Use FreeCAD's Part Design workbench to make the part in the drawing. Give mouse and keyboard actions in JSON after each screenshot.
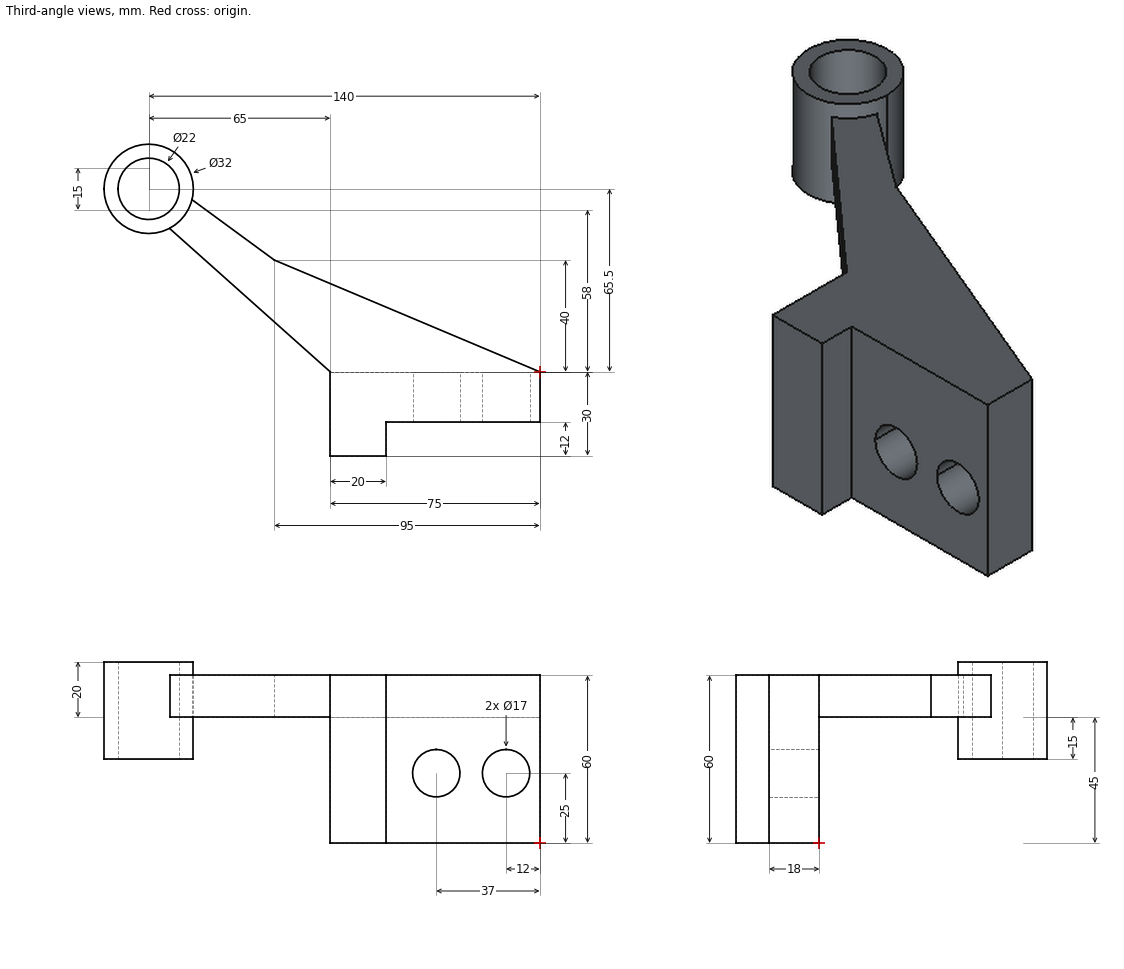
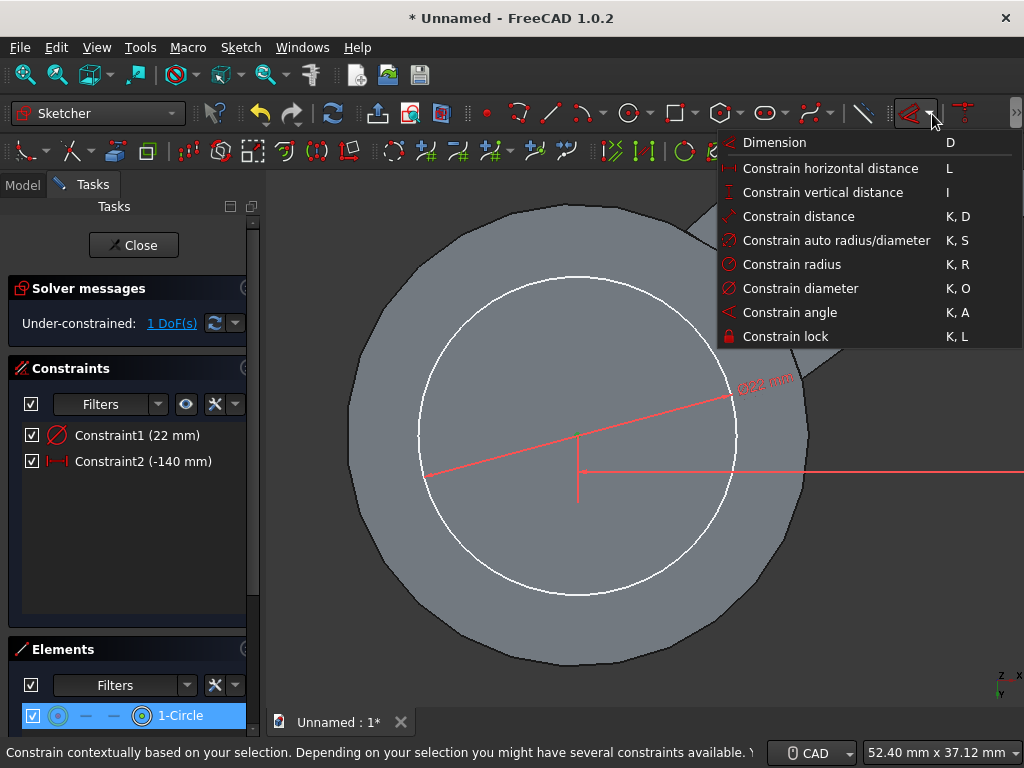
{"action": "left_click", "coordinate": [870, 192]}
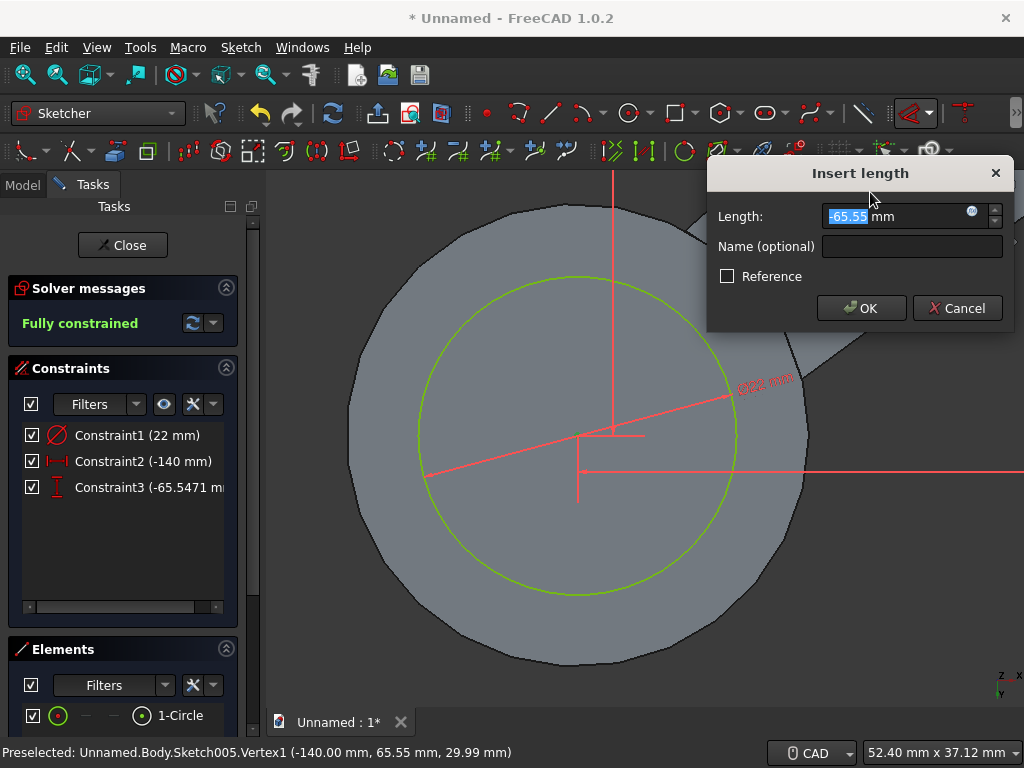
{"action": "type", "text": "-65.5"}
{"action": "key", "text": "Return"}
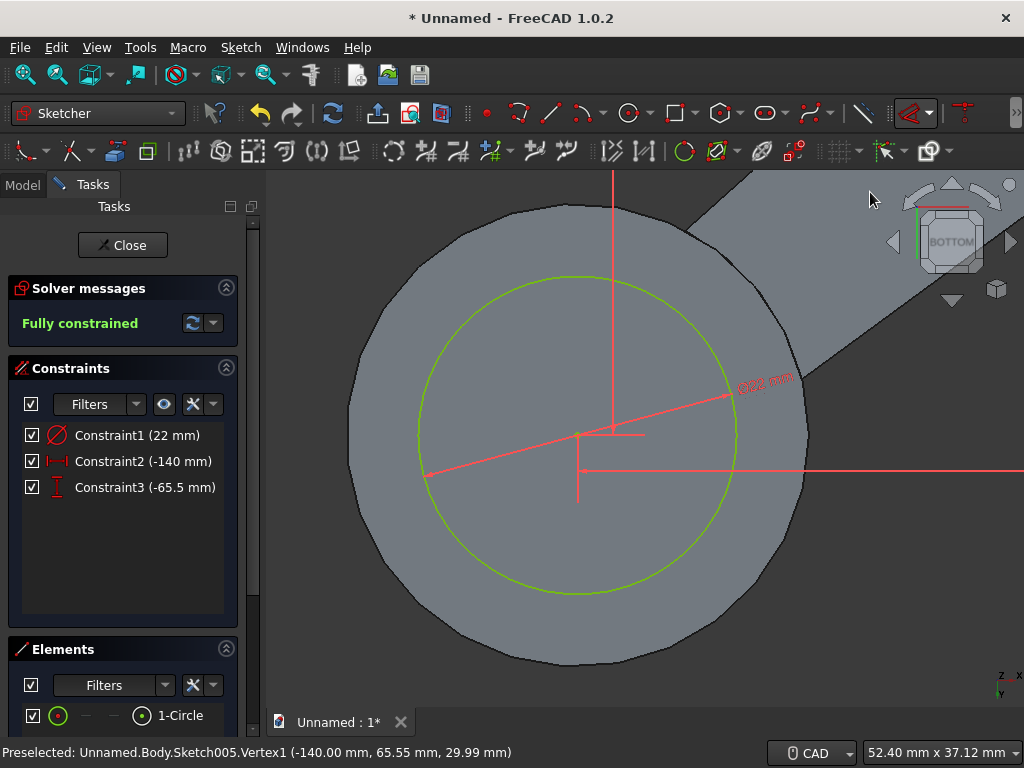
{"action": "left_click", "coordinate": [123, 245]}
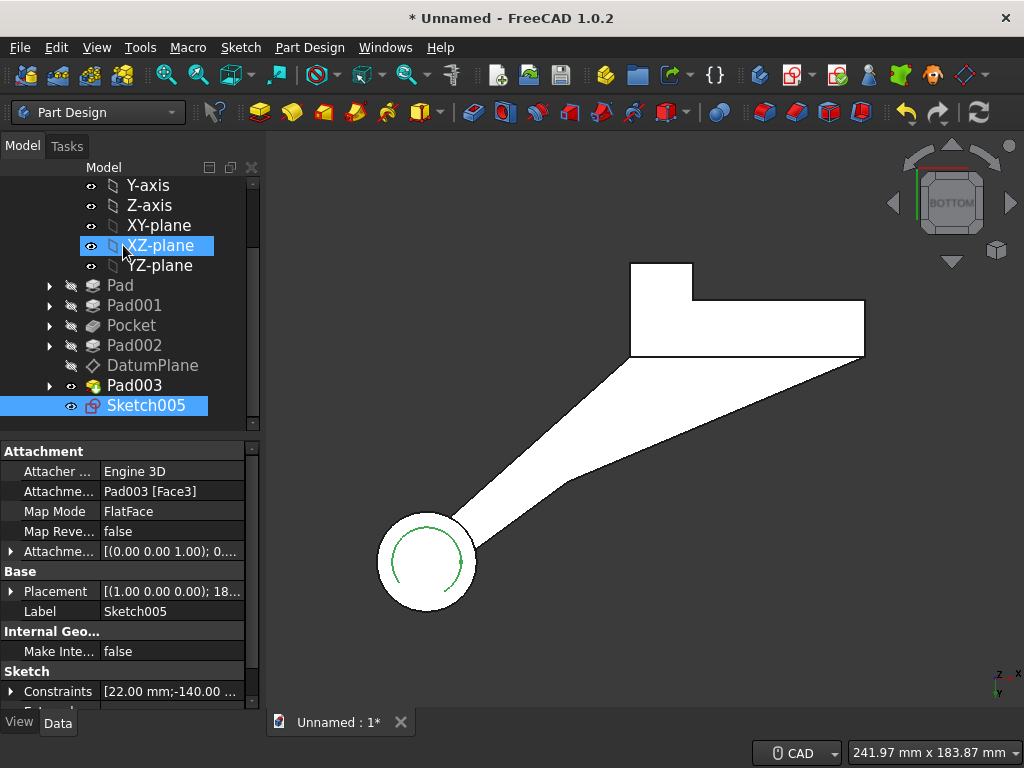
{"action": "left_click", "coordinate": [474, 112]}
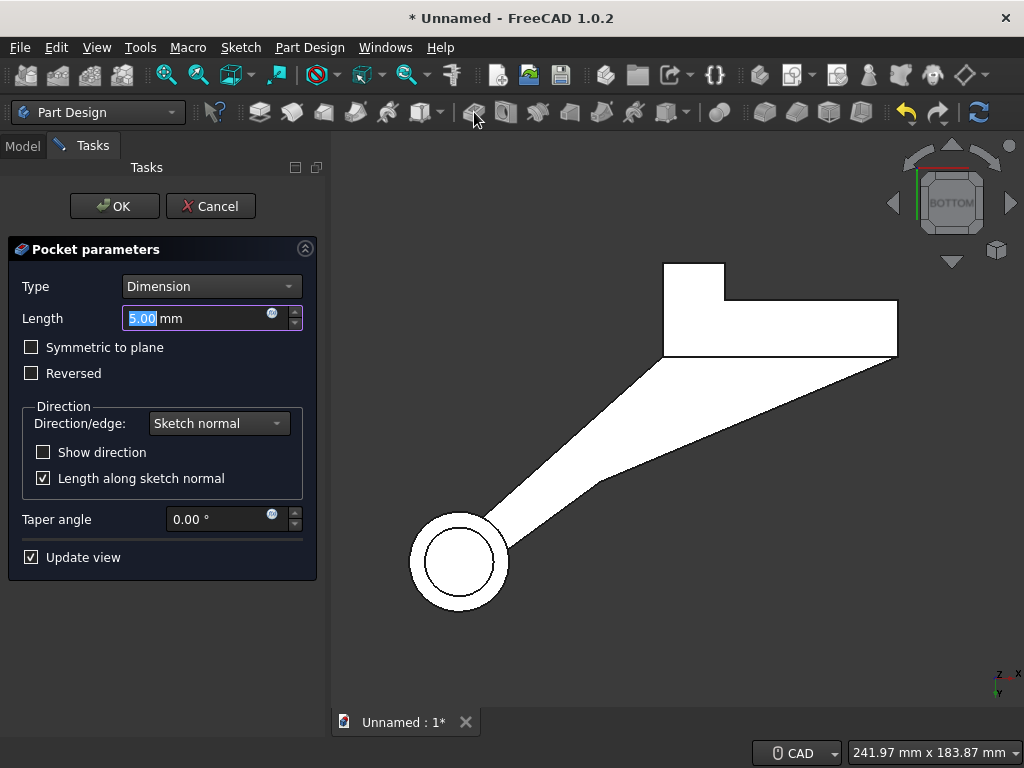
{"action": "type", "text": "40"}
{"action": "key", "text": "Tab"}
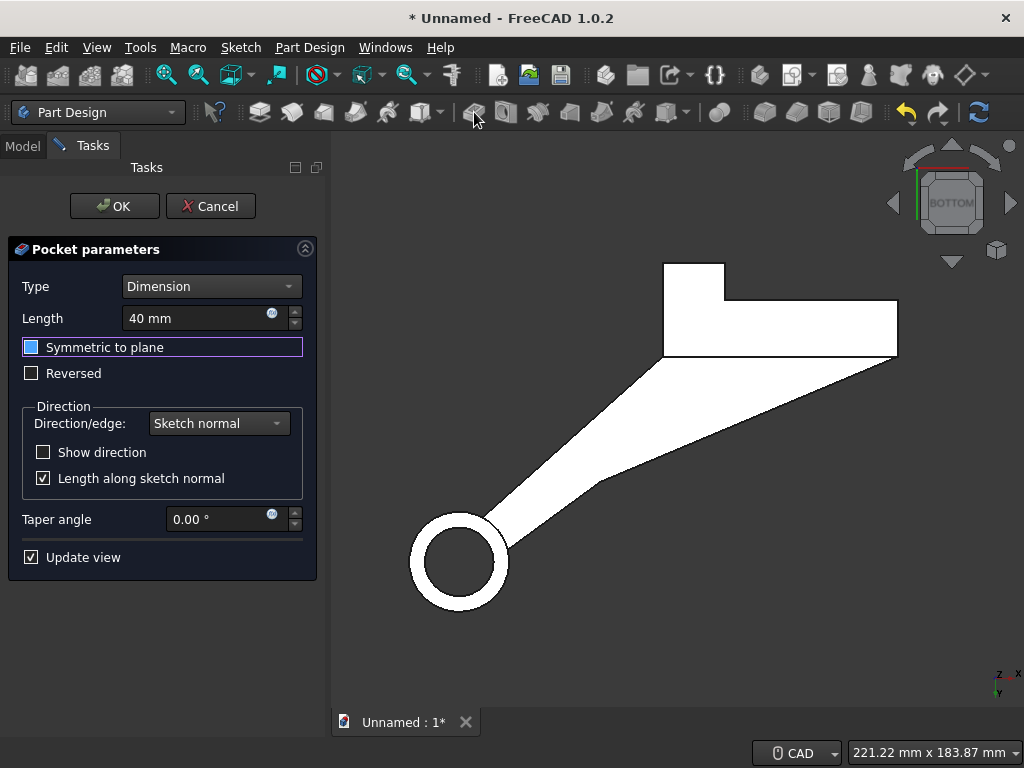
{"action": "left_click", "coordinate": [115, 206]}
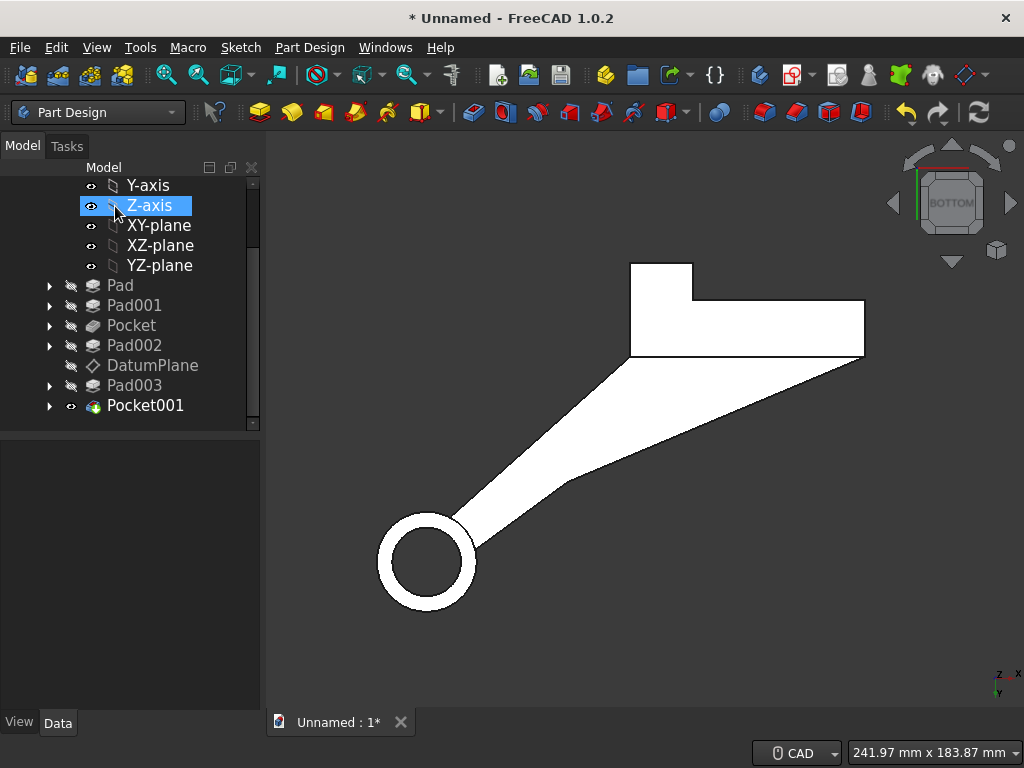
{"action": "key", "text": "4"}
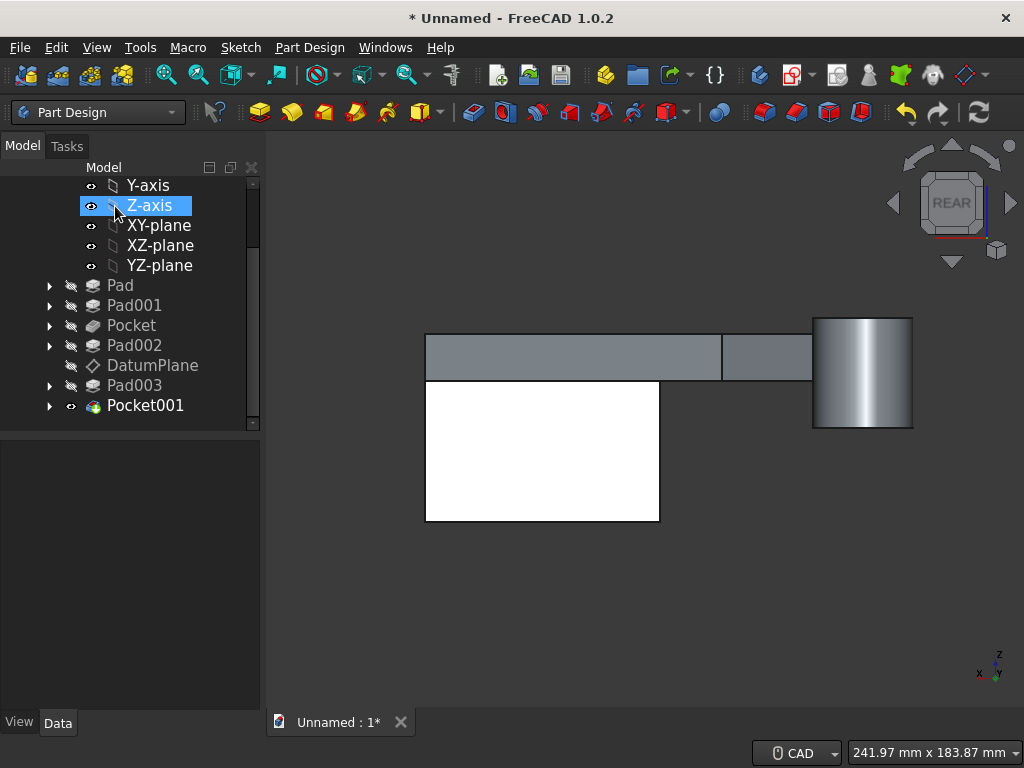
{"action": "left_click", "coordinate": [509, 450]}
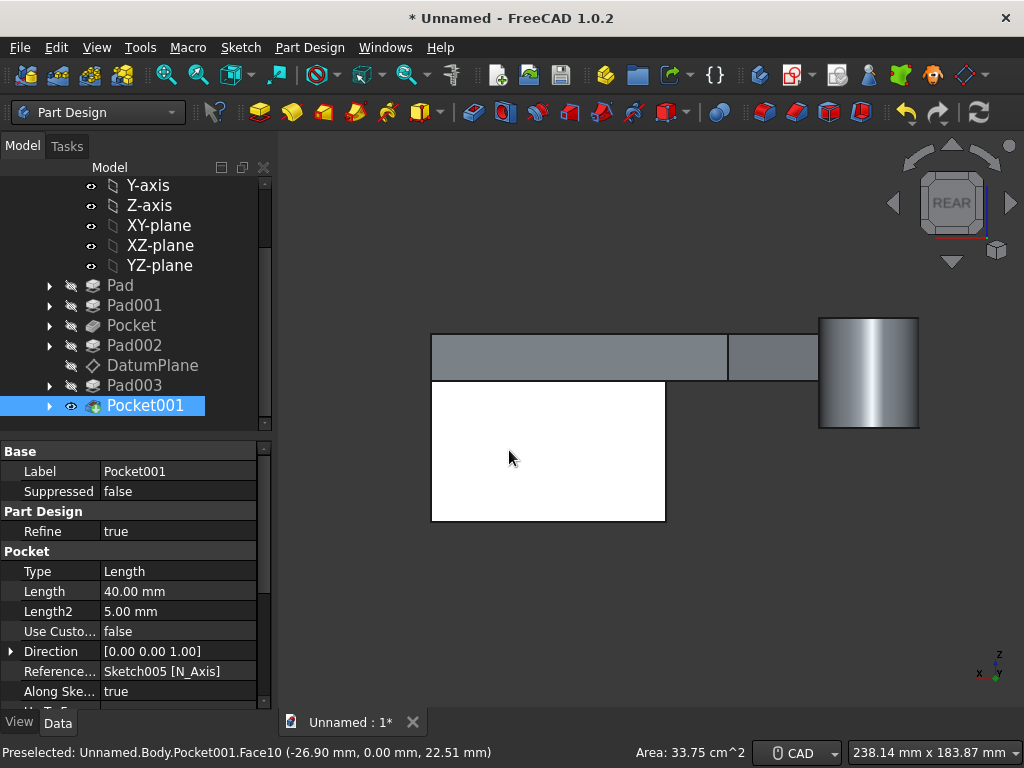
{"action": "left_click", "coordinate": [792, 76]}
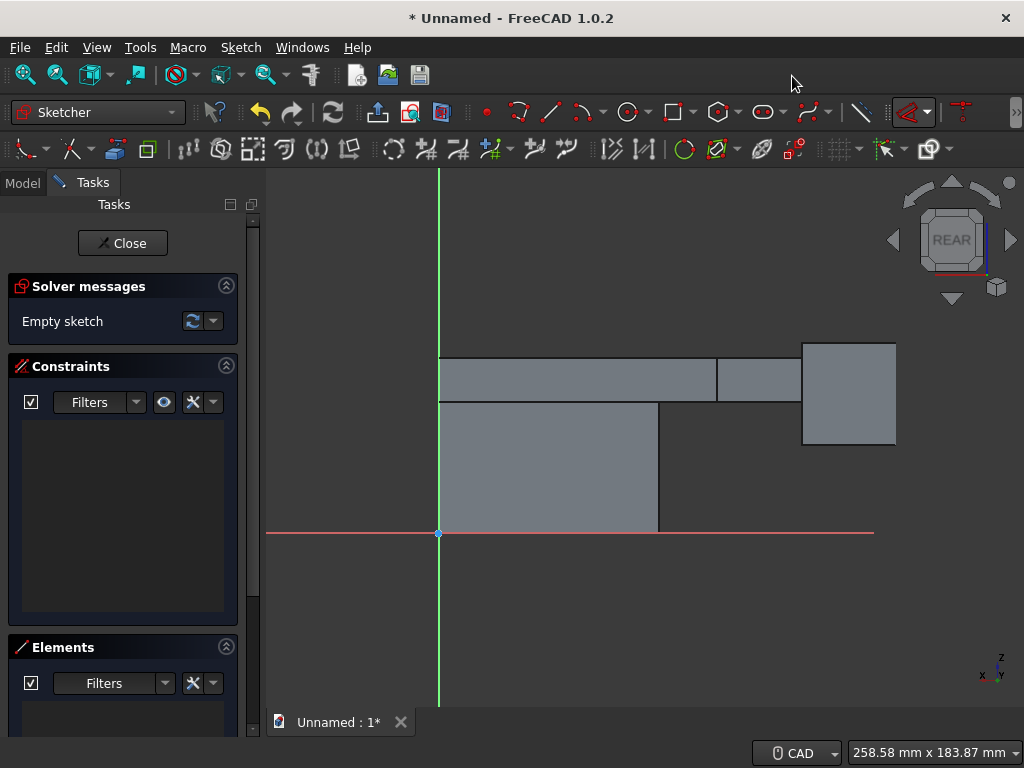
{"action": "left_click", "coordinate": [442, 112]}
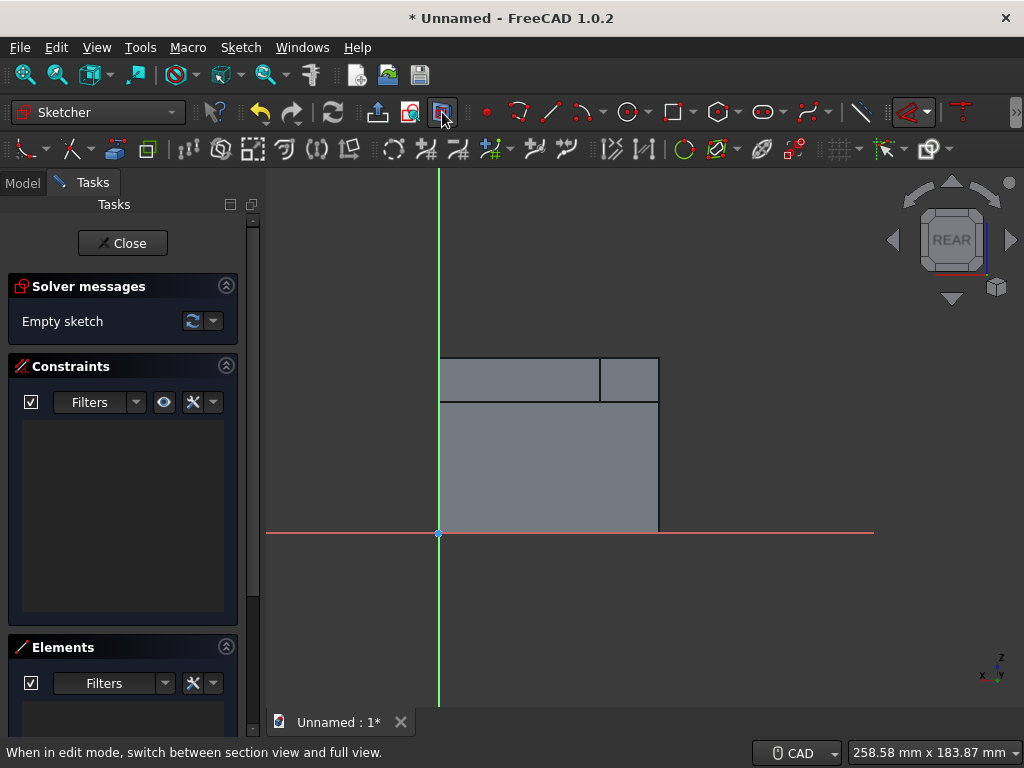
{"action": "scroll", "coordinate": [464, 512], "scroll_direction": "up", "scroll_amount": 5}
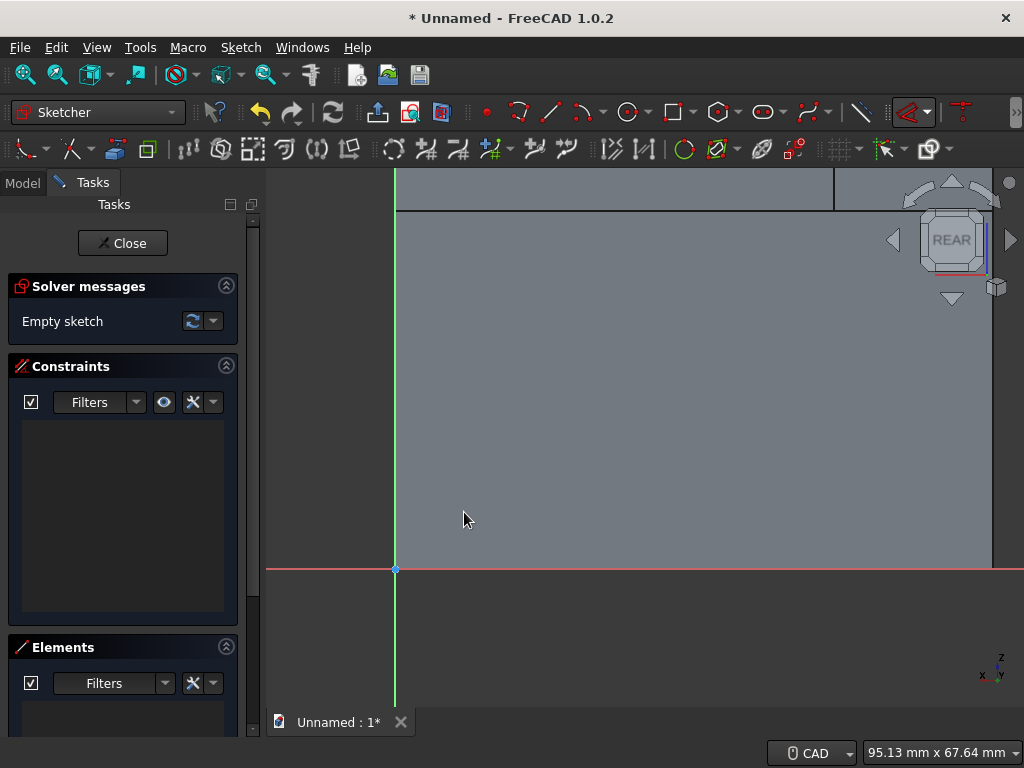
{"action": "left_click", "coordinate": [628, 112]}